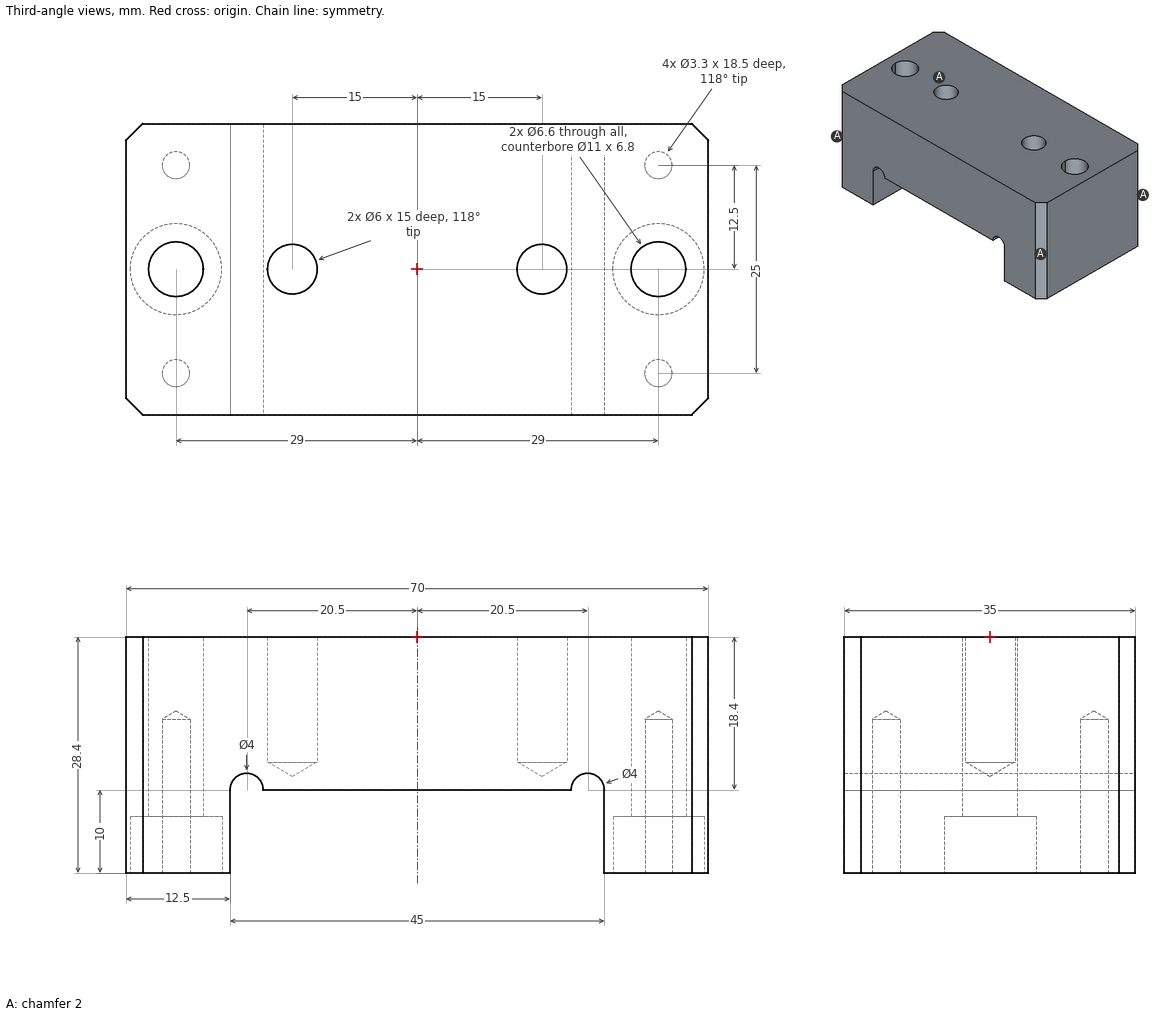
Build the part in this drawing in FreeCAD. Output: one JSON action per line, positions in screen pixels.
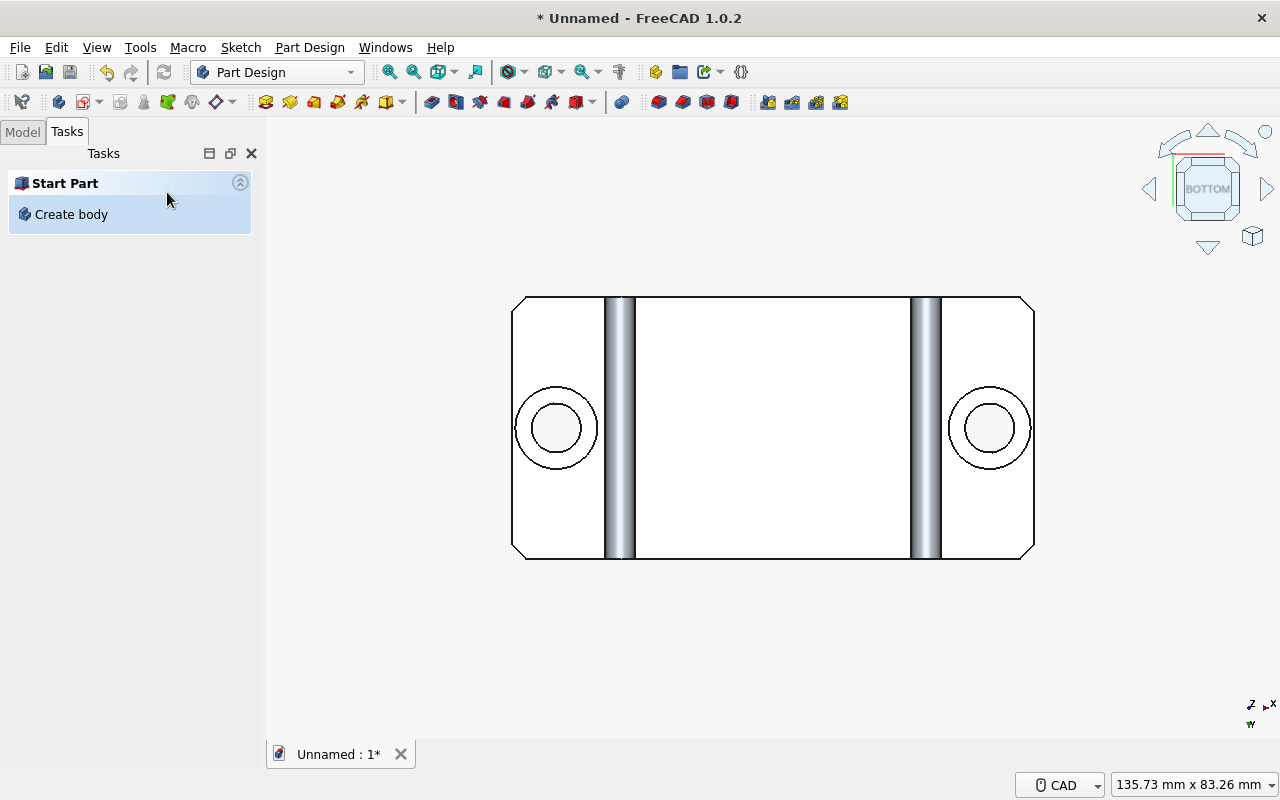
{"action": "left_click", "coordinate": [558, 352]}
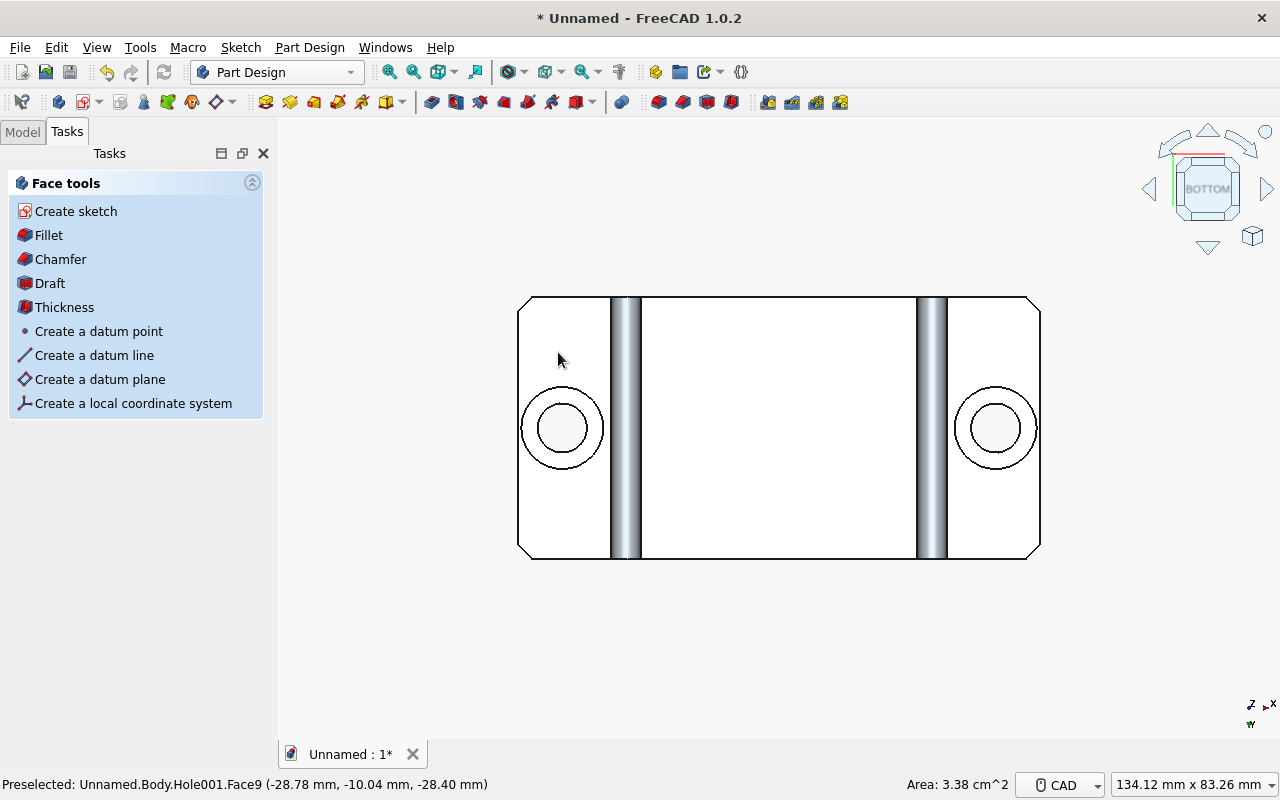
{"action": "left_click", "coordinate": [84, 102]}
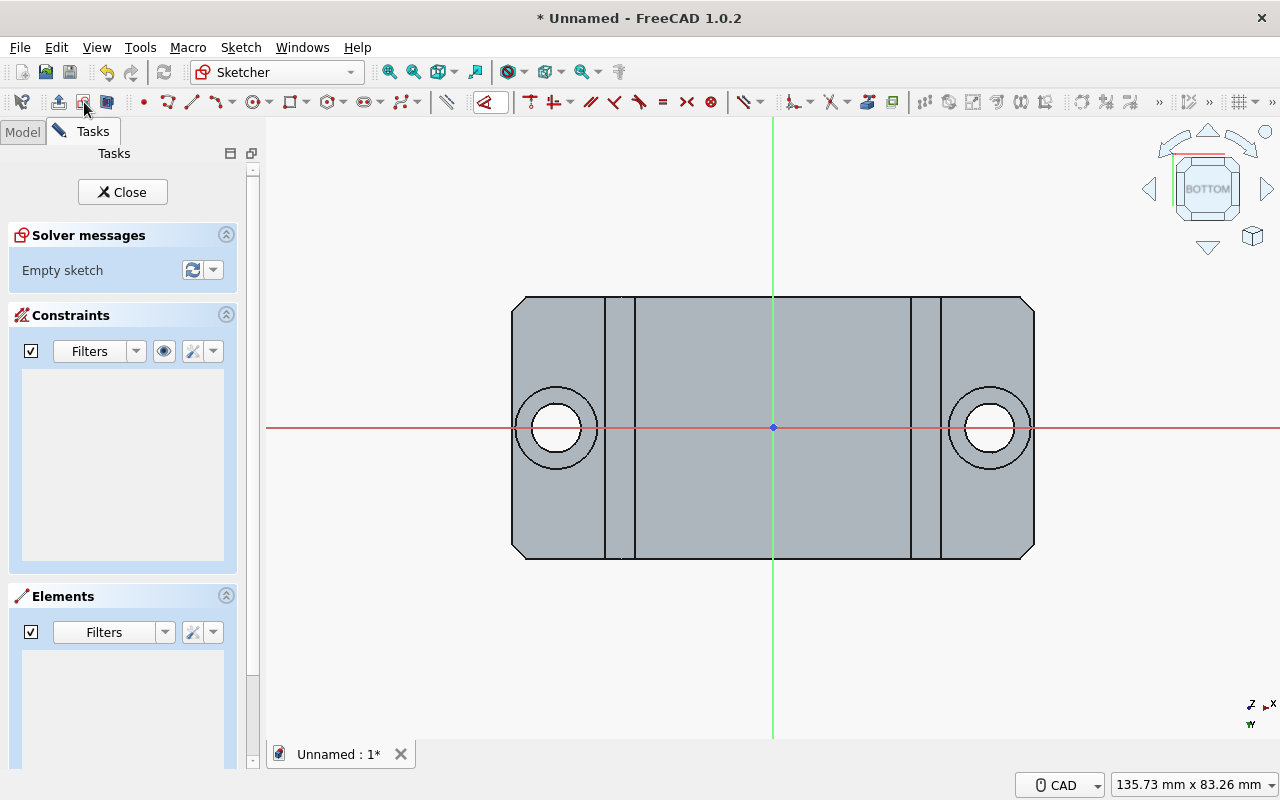
{"action": "key", "text": "g c"}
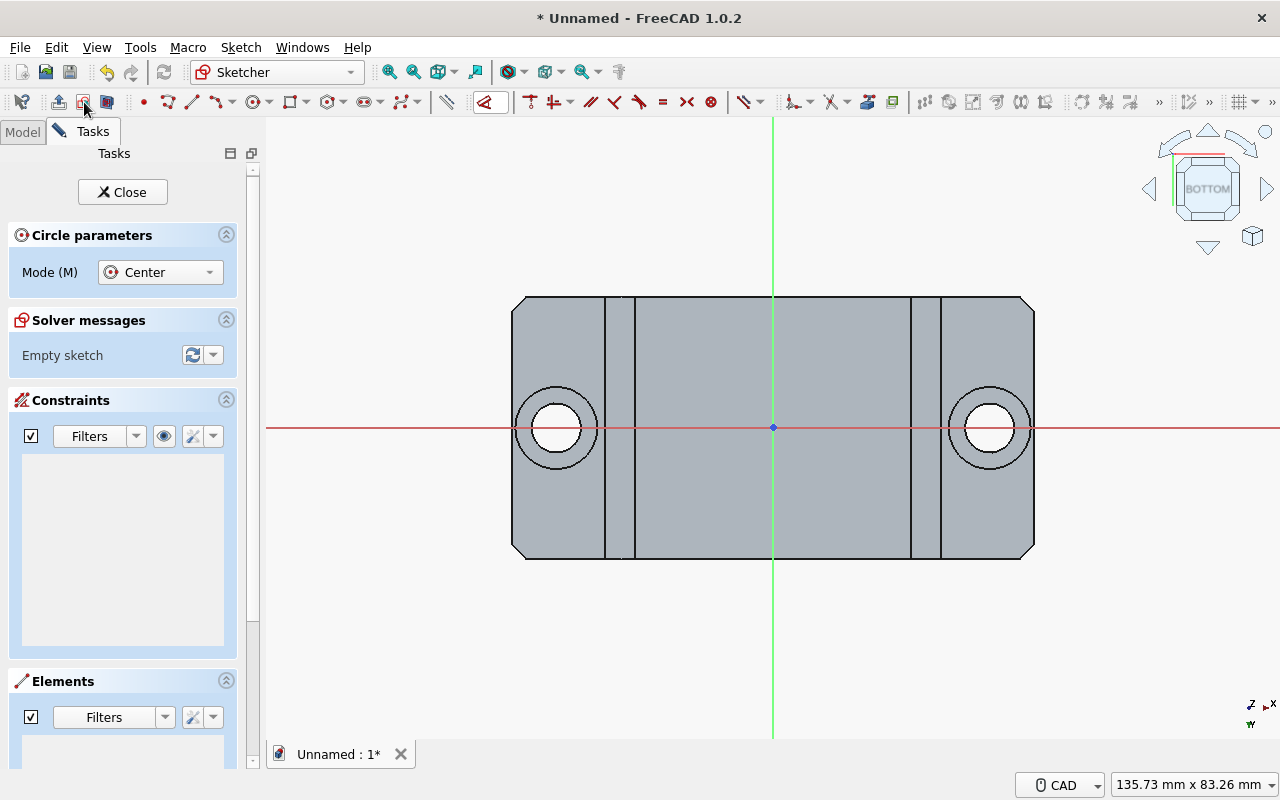
{"action": "scroll", "coordinate": [990, 521], "scroll_direction": "up", "scroll_amount": 4}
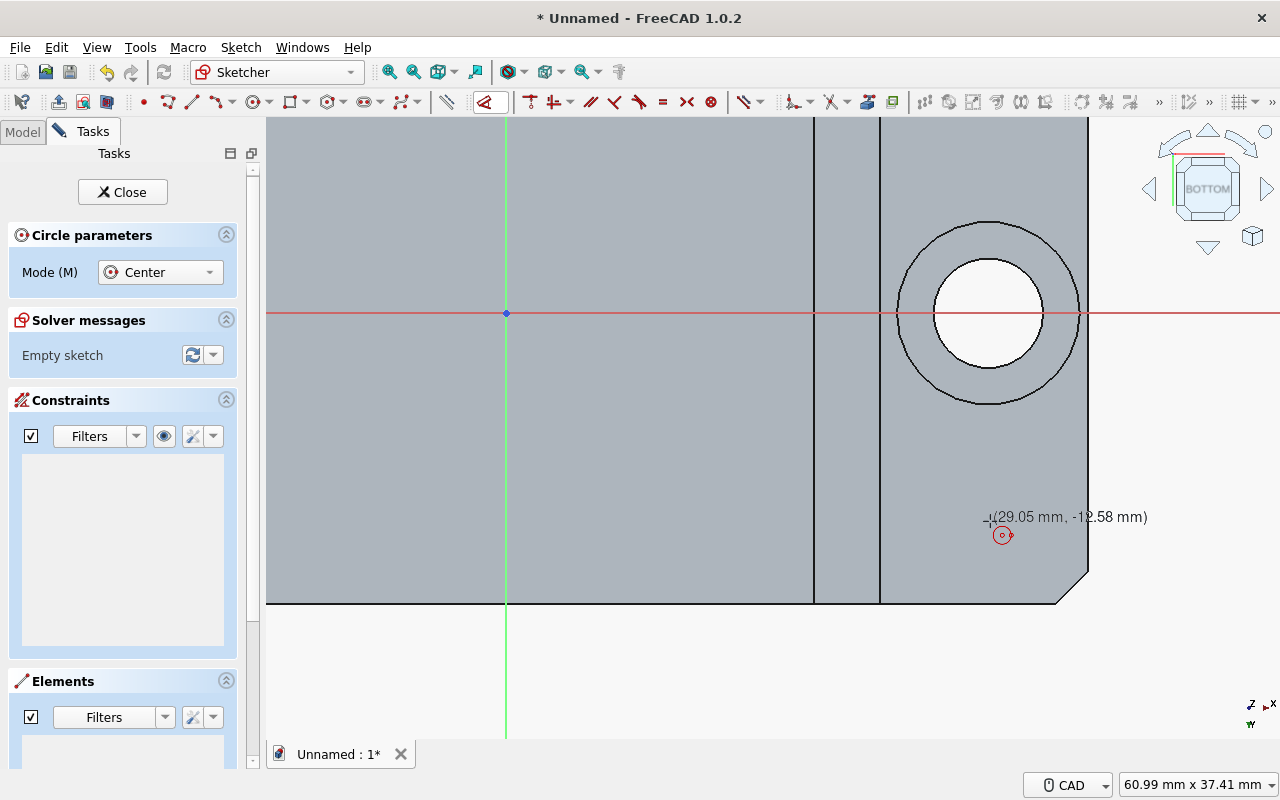
{"action": "left_click", "coordinate": [988, 521]}
{"action": "left_click", "coordinate": [1008, 502]}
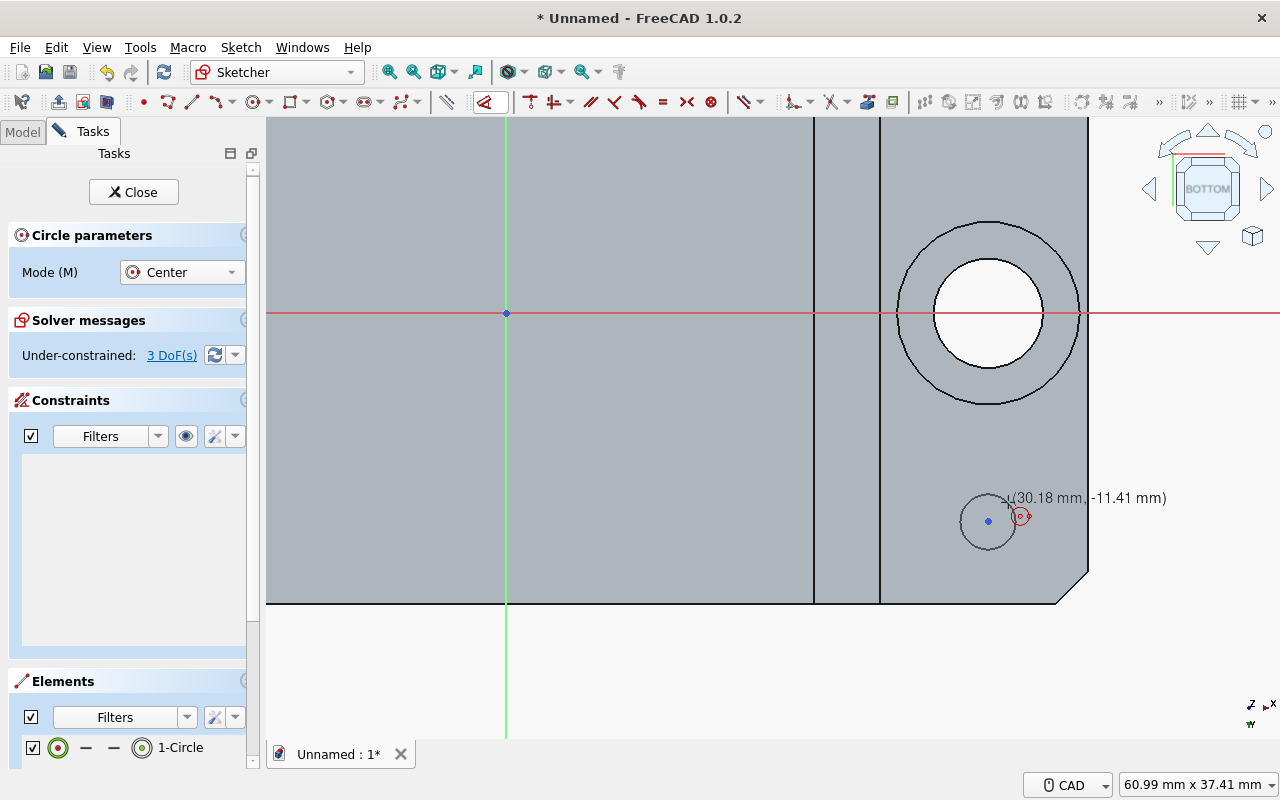
{"action": "scroll", "coordinate": [946, 568], "scroll_direction": "down", "scroll_amount": 3}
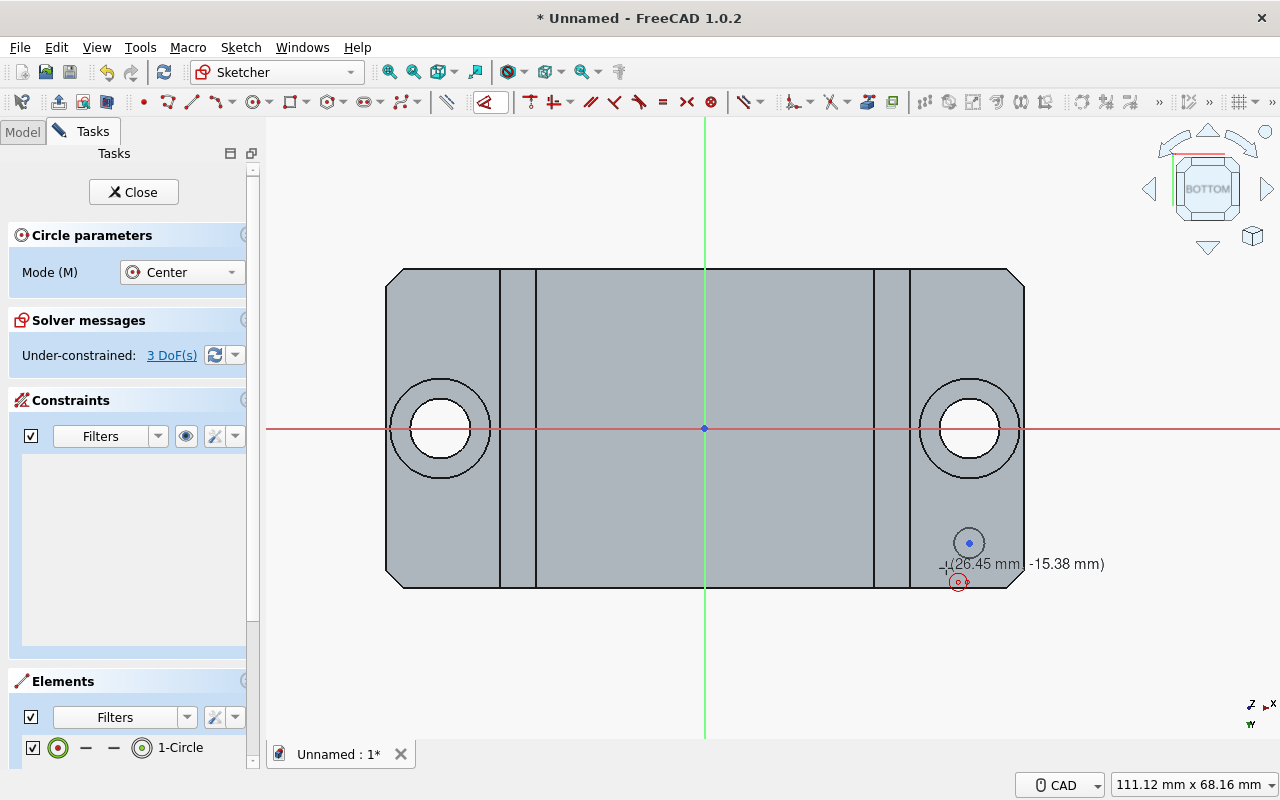
{"action": "scroll", "coordinate": [970, 314], "scroll_direction": "up", "scroll_amount": 3}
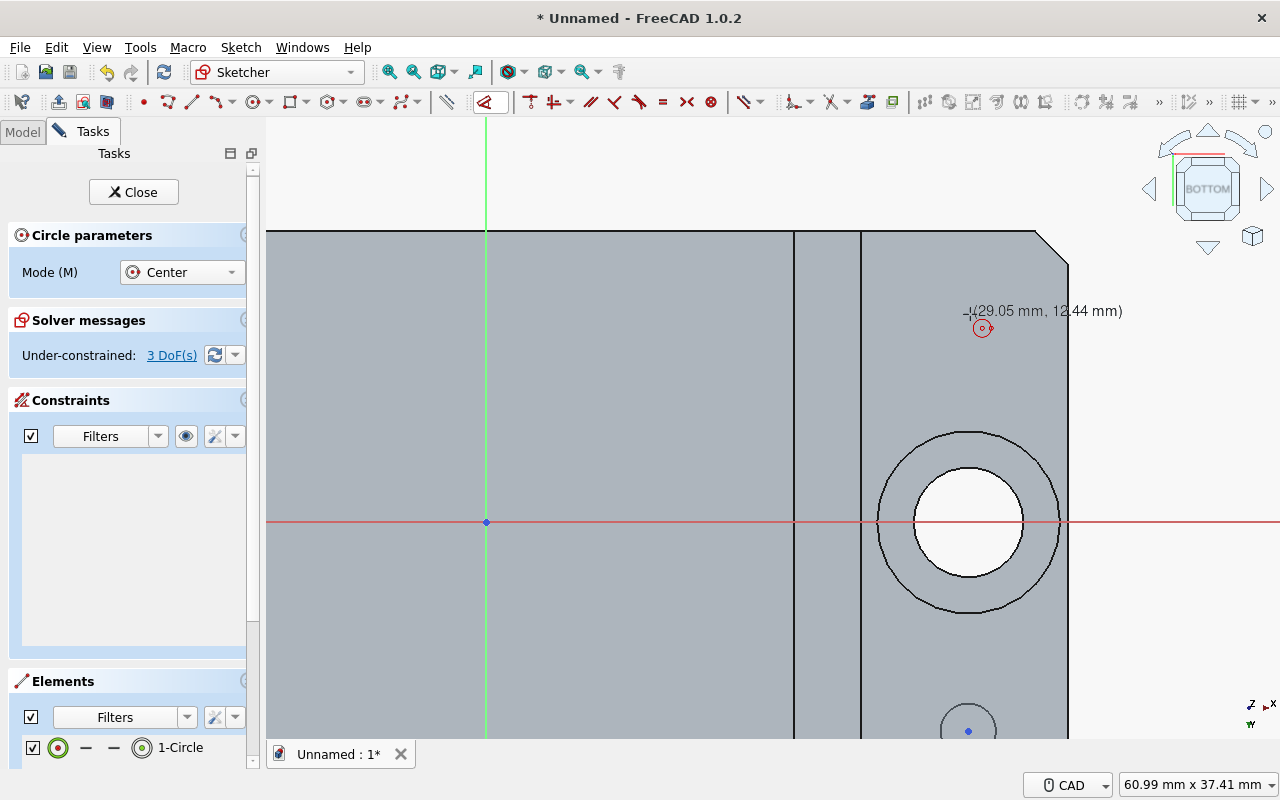
{"action": "left_click", "coordinate": [969, 315]}
{"action": "left_click", "coordinate": [988, 295]}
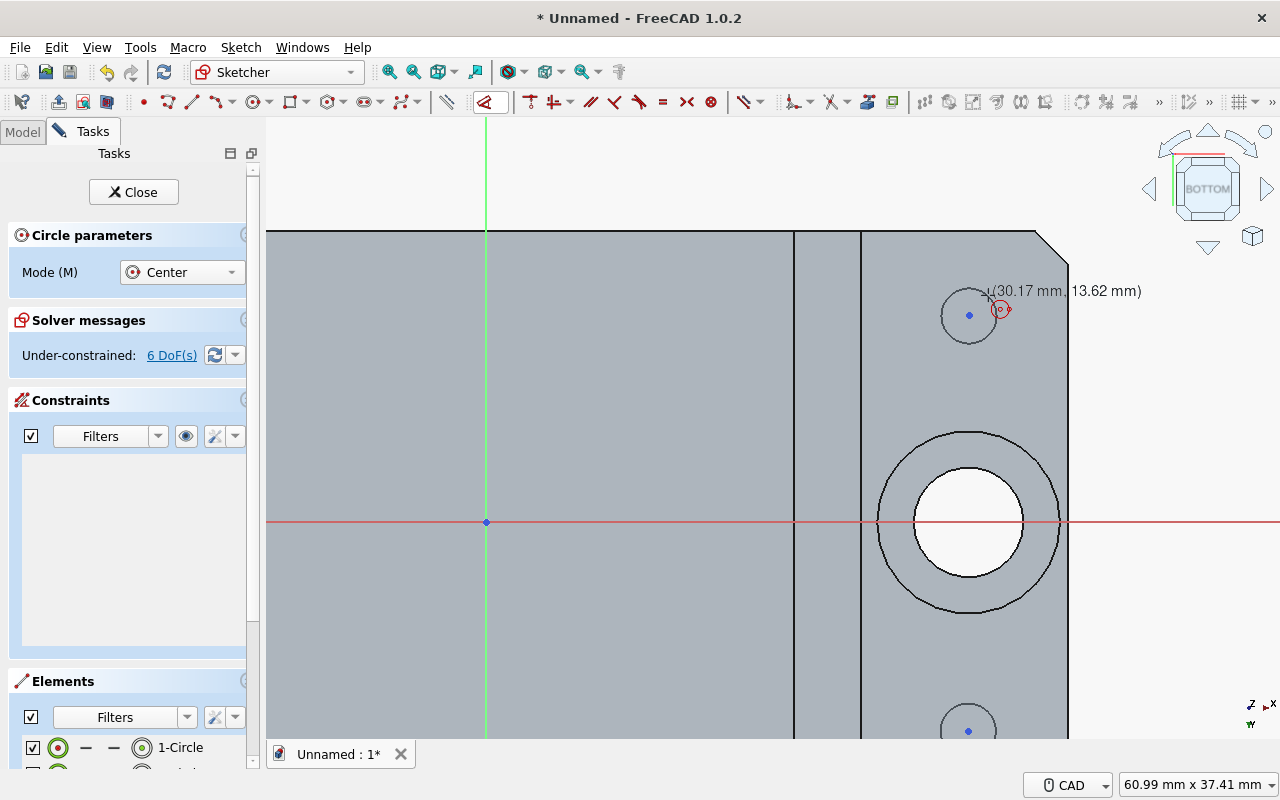
{"action": "scroll", "coordinate": [970, 313], "scroll_direction": "down", "scroll_amount": 3}